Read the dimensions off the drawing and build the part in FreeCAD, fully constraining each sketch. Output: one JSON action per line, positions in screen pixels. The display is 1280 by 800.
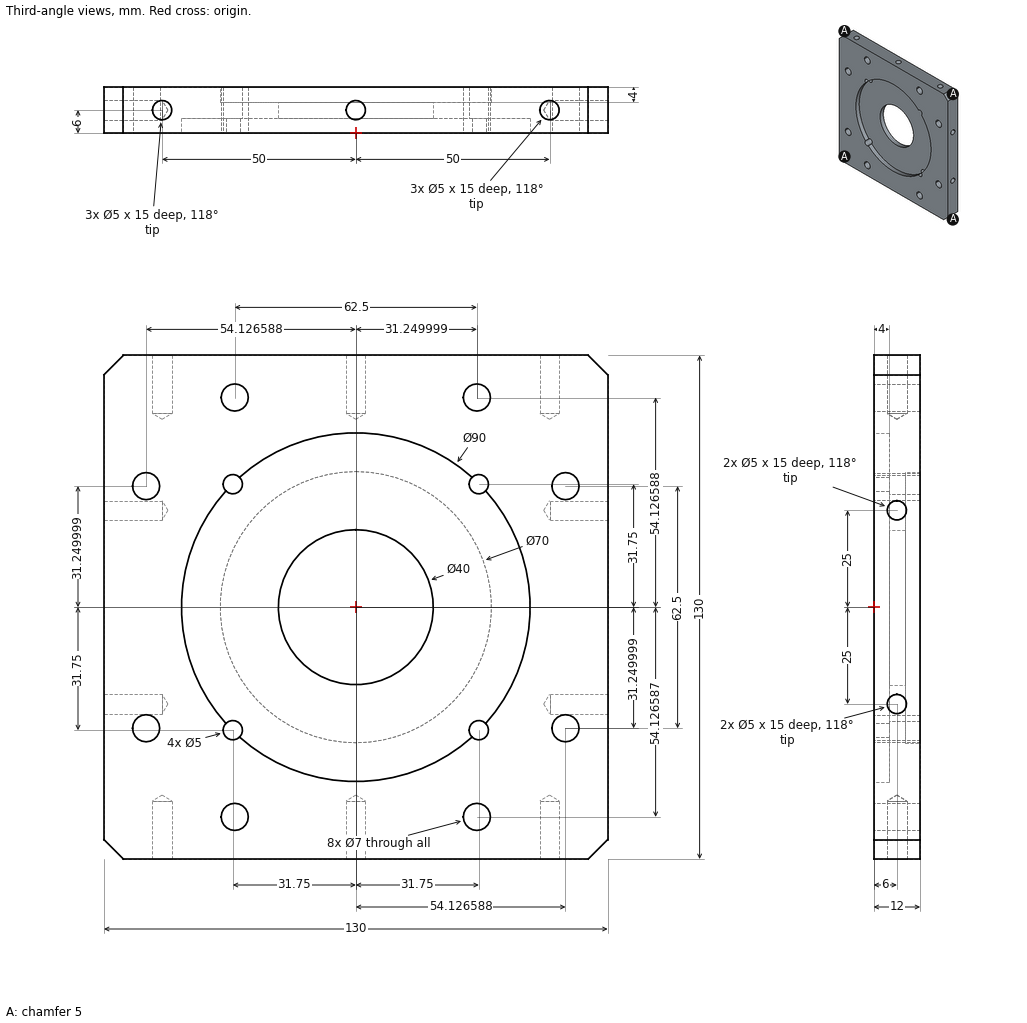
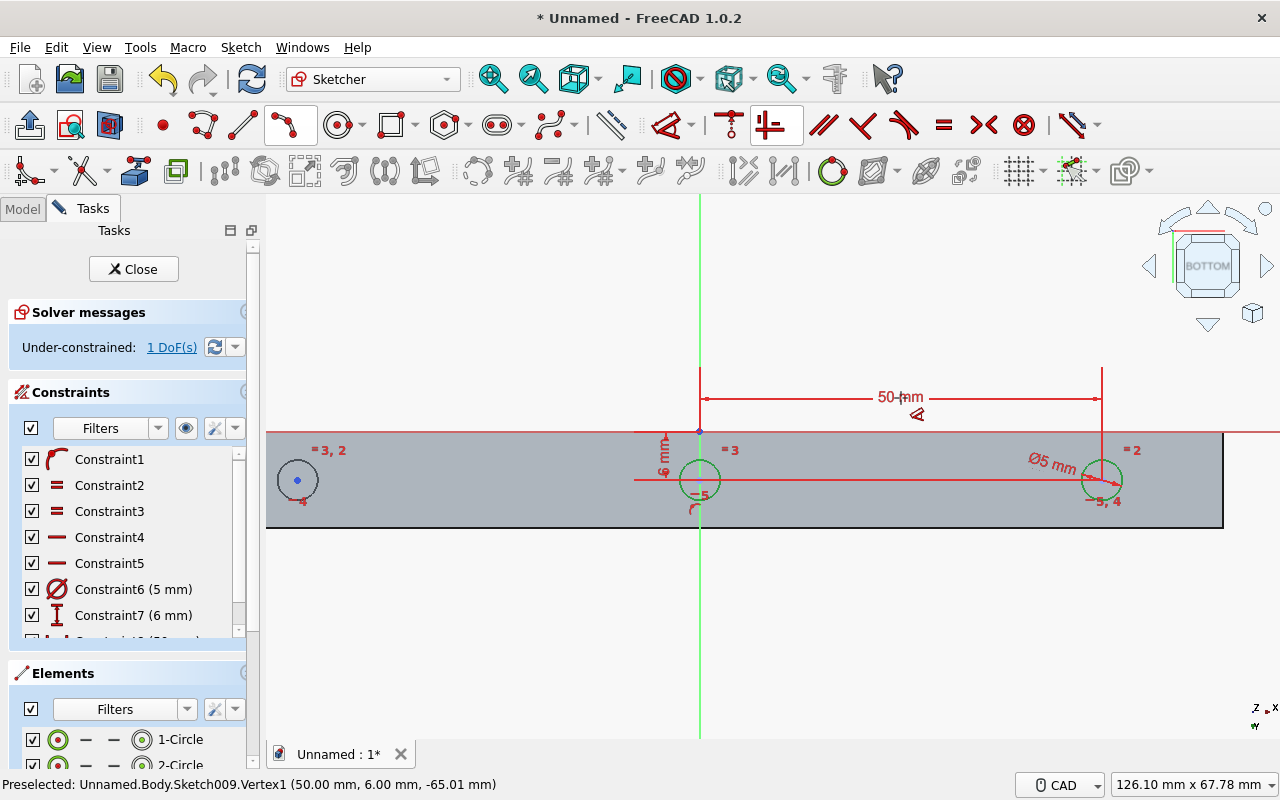
{"action": "left_click", "coordinate": [298, 480]}
{"action": "left_click", "coordinate": [499, 398]}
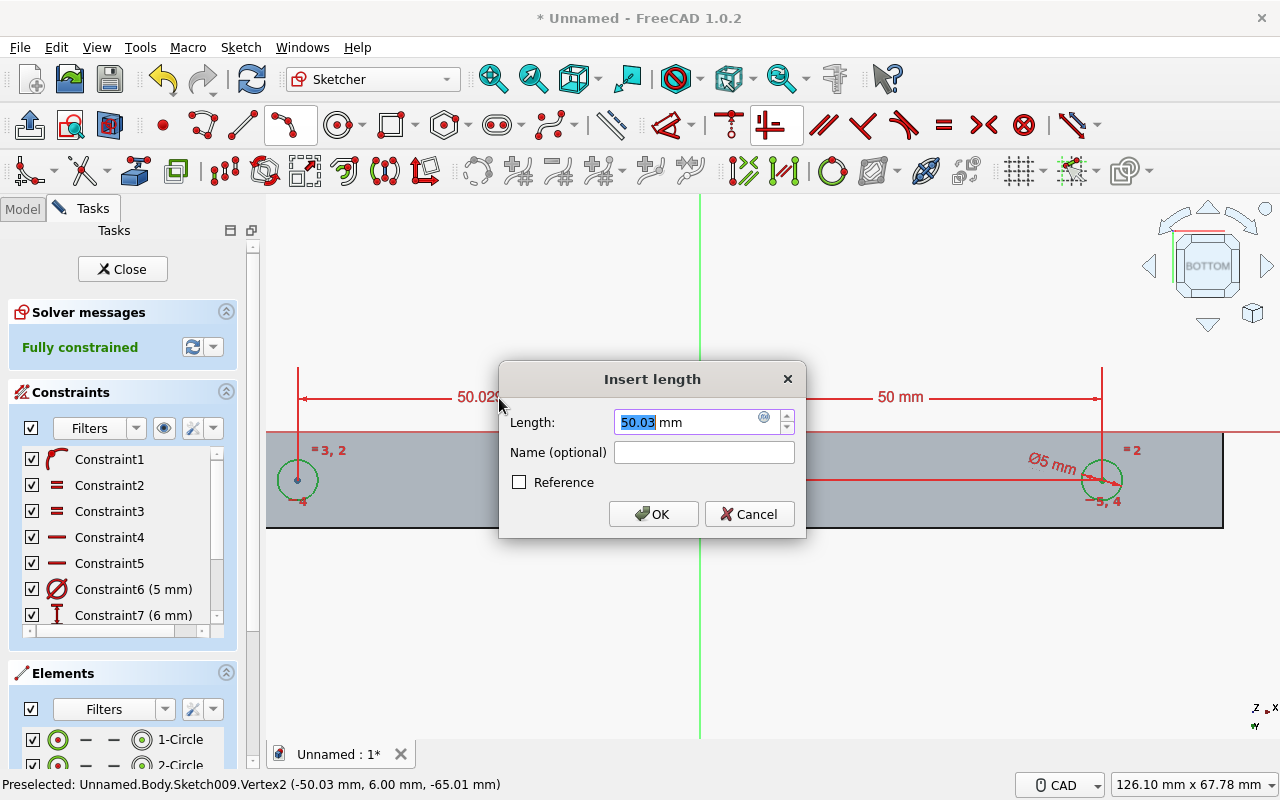
{"action": "type", "text": "50"}
{"action": "key", "text": "Return"}
{"action": "key", "text": "Escape"}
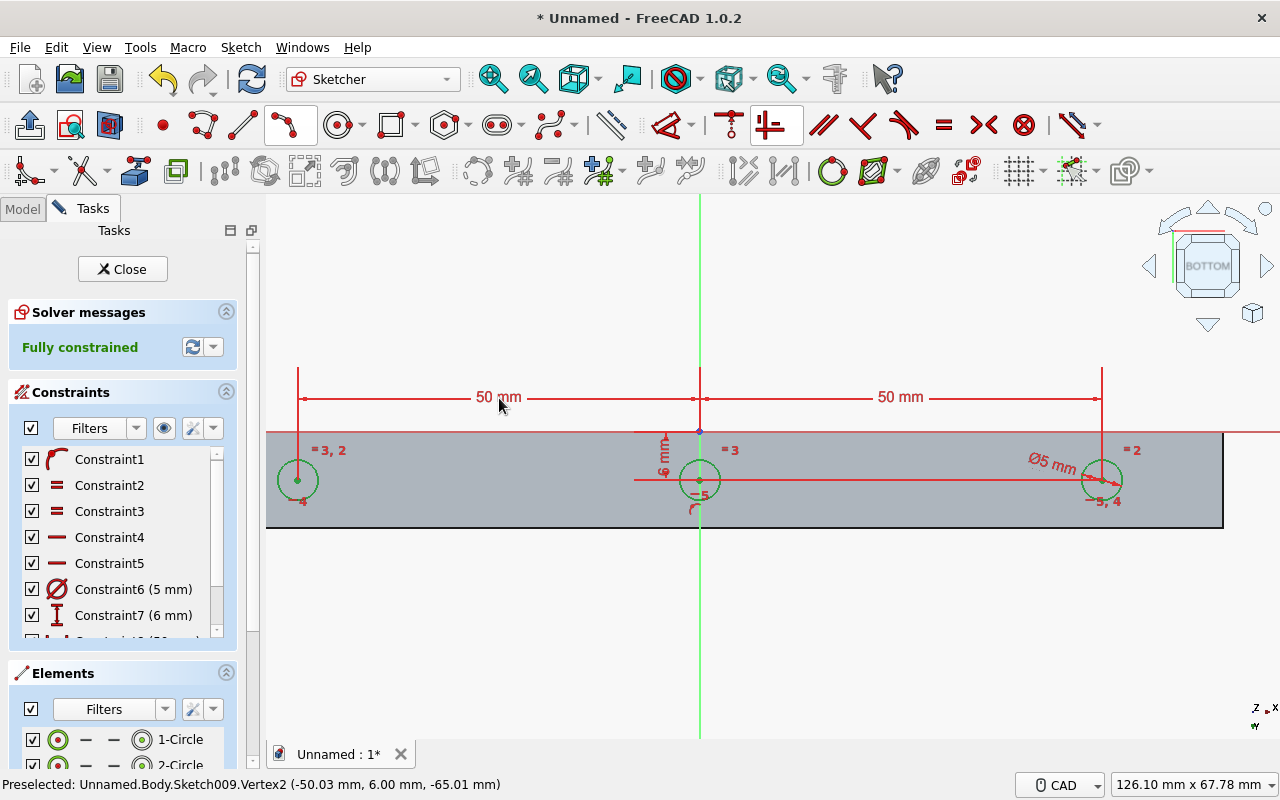
{"action": "left_click", "coordinate": [123, 269]}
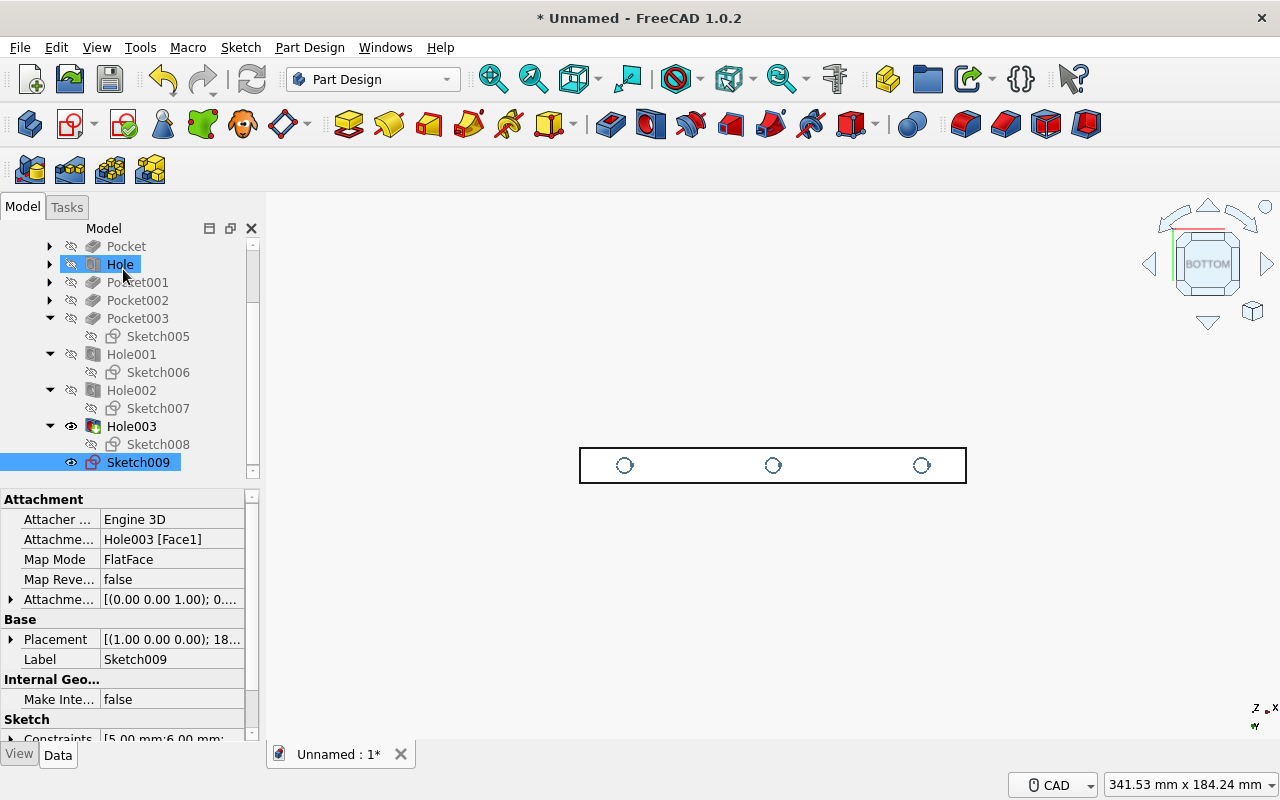
{"action": "left_click", "coordinate": [652, 124]}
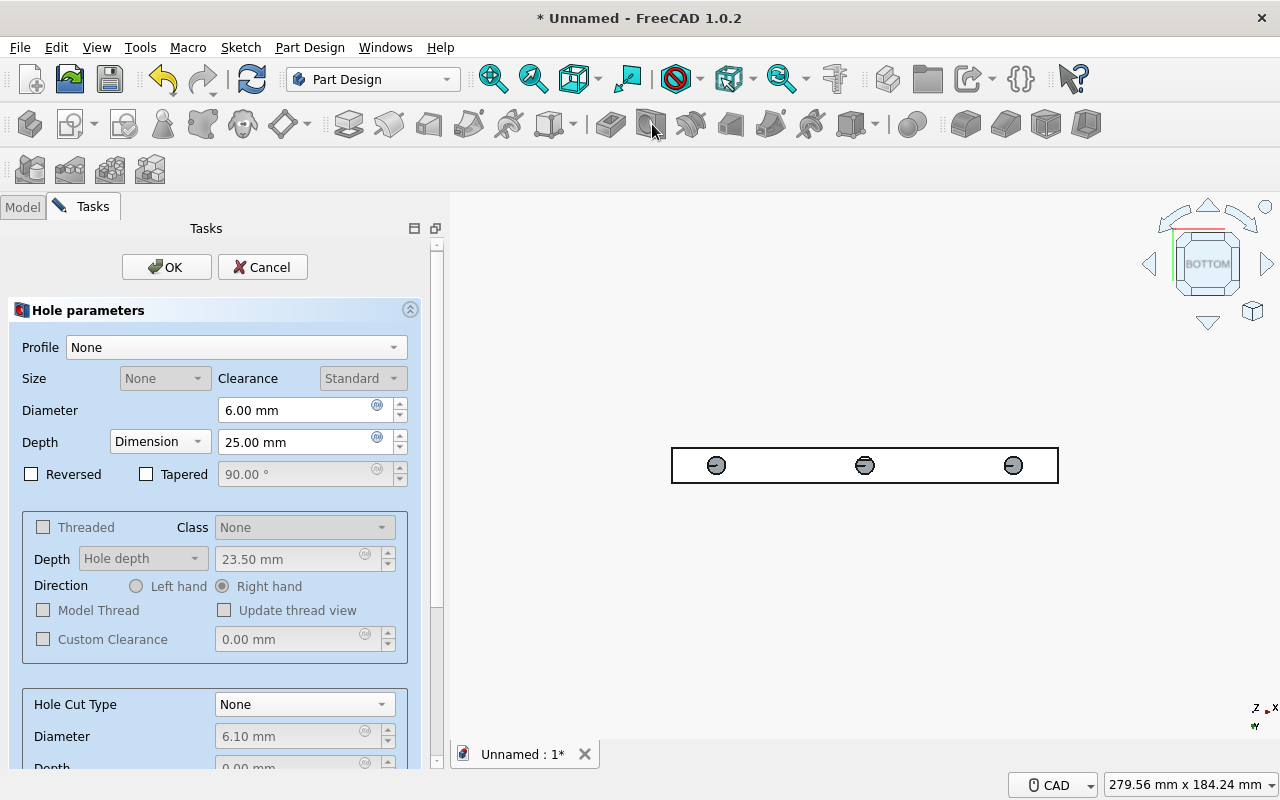
{"action": "triple_click", "coordinate": [305, 410]}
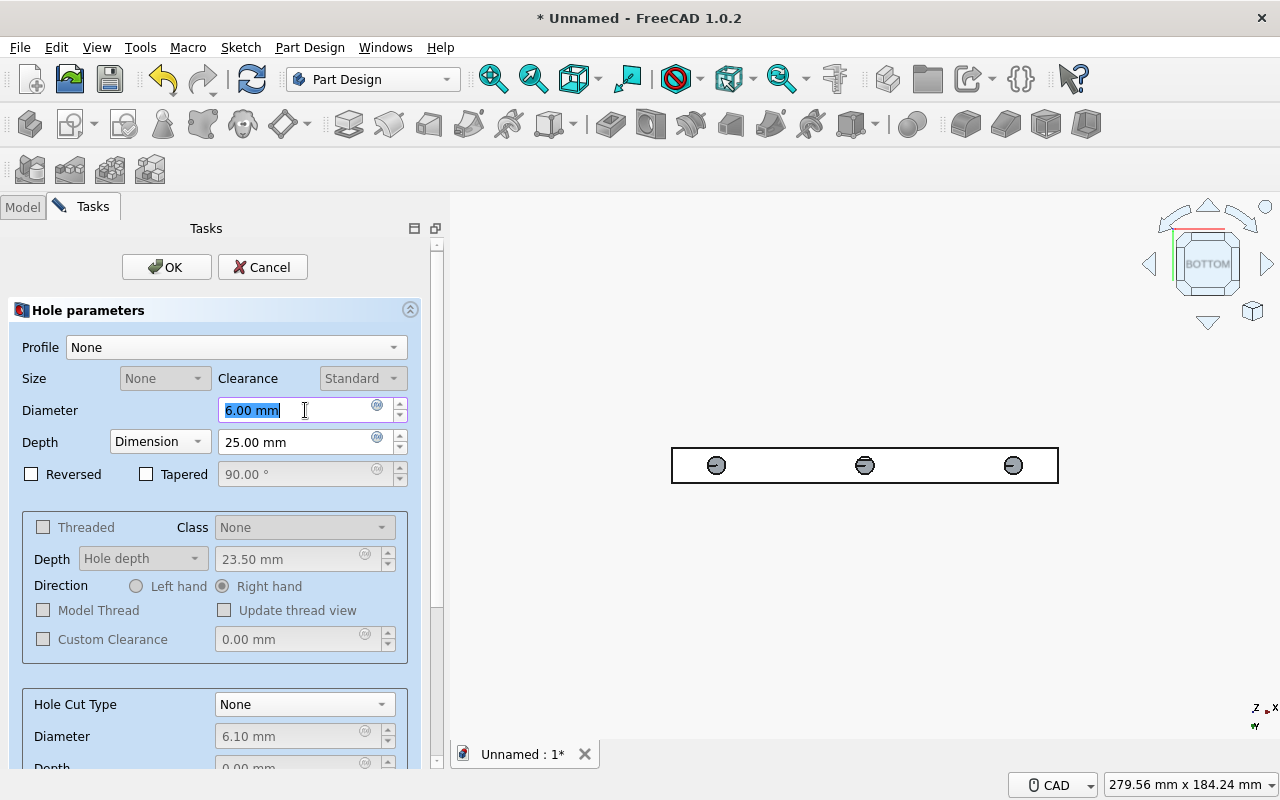
{"action": "type", "text": "5"}
{"action": "key", "text": "Tab"}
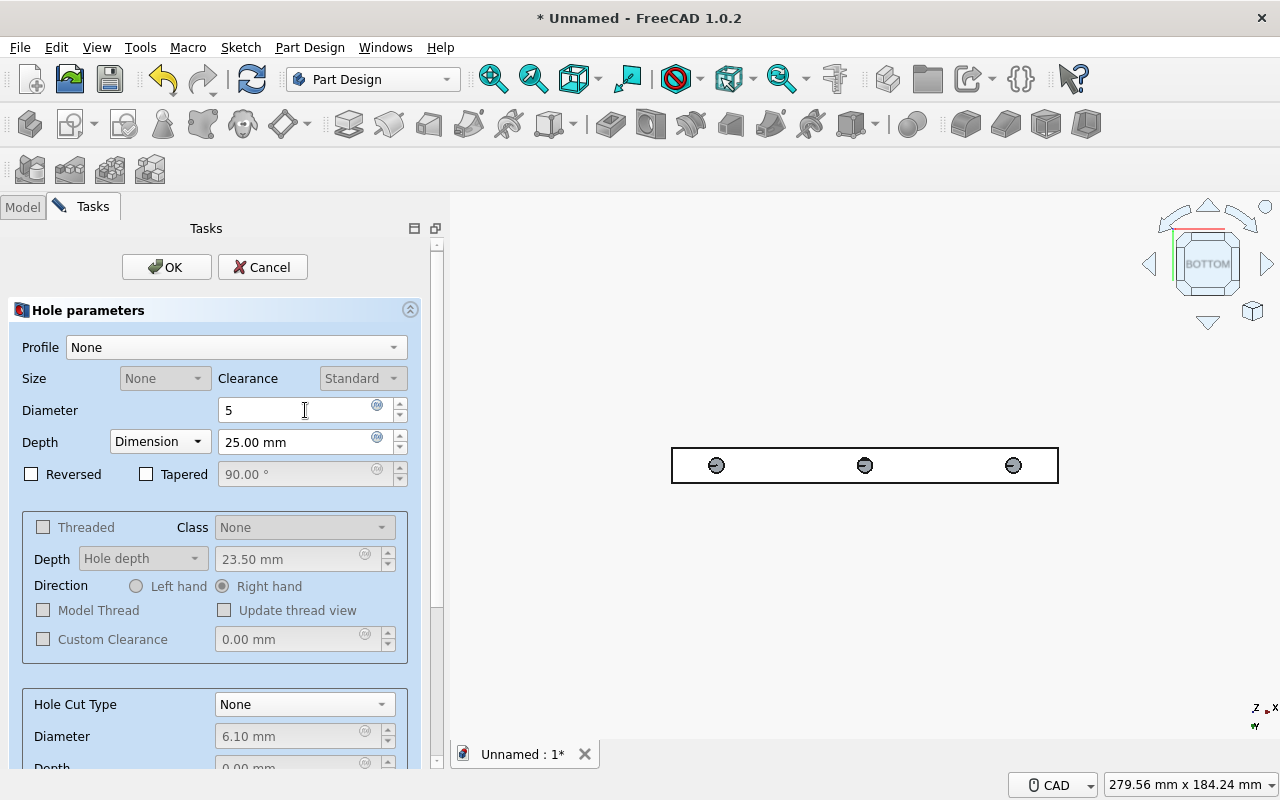
{"action": "triple_click", "coordinate": [305, 442]}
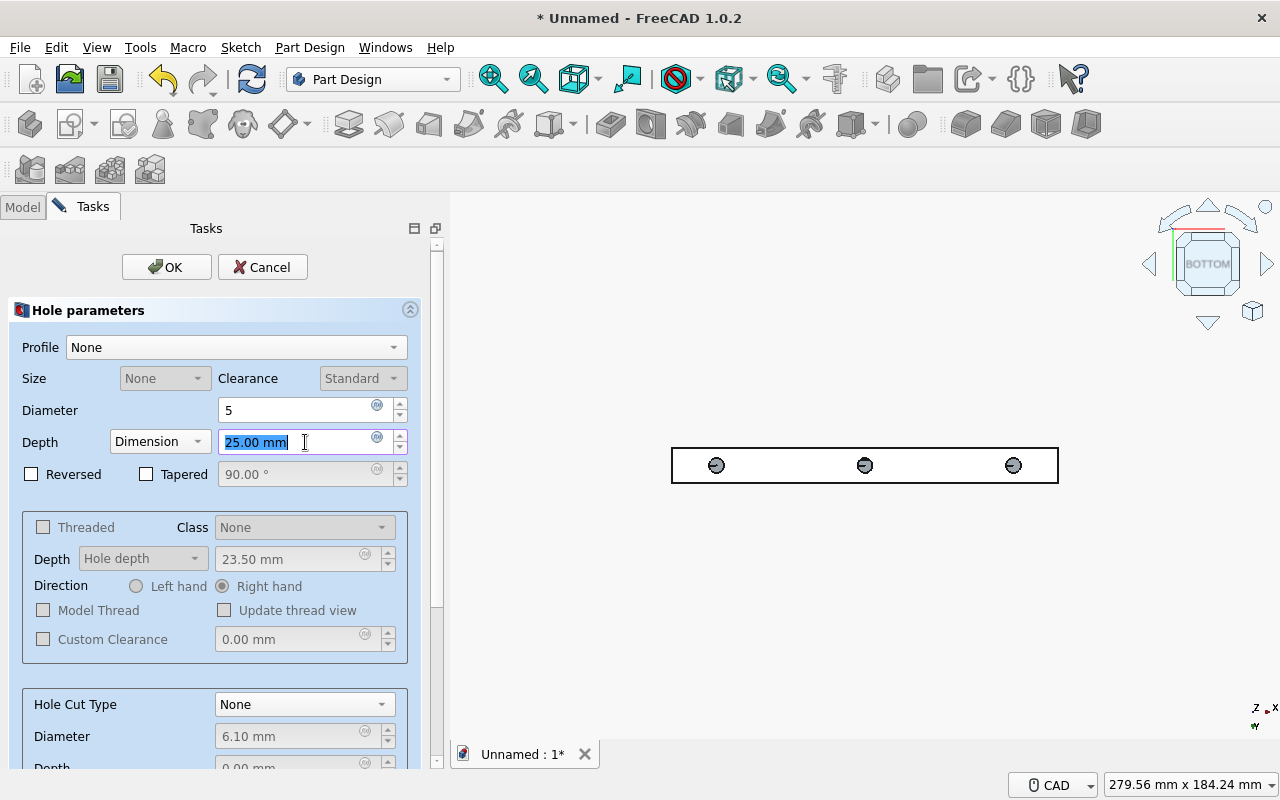
{"action": "type", "text": "15"}
{"action": "key", "text": "Tab"}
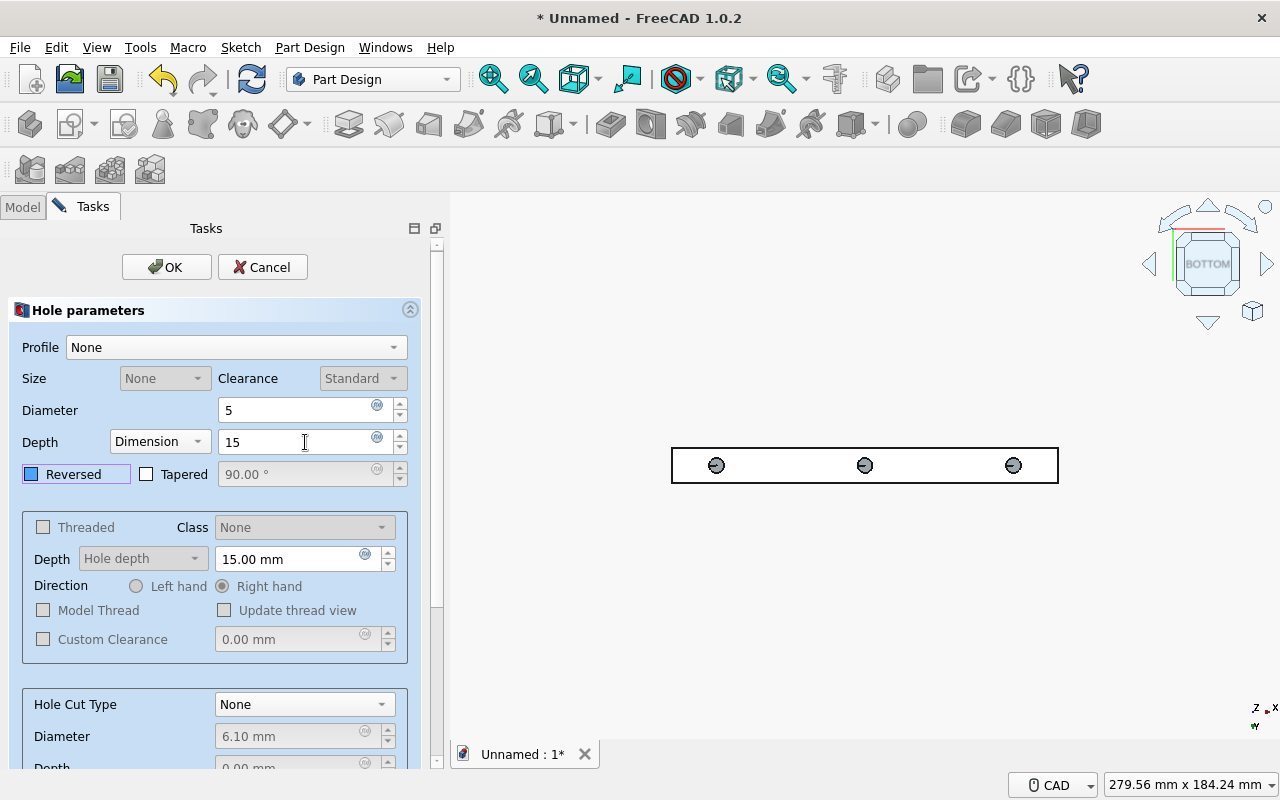
{"action": "left_click", "coordinate": [167, 267]}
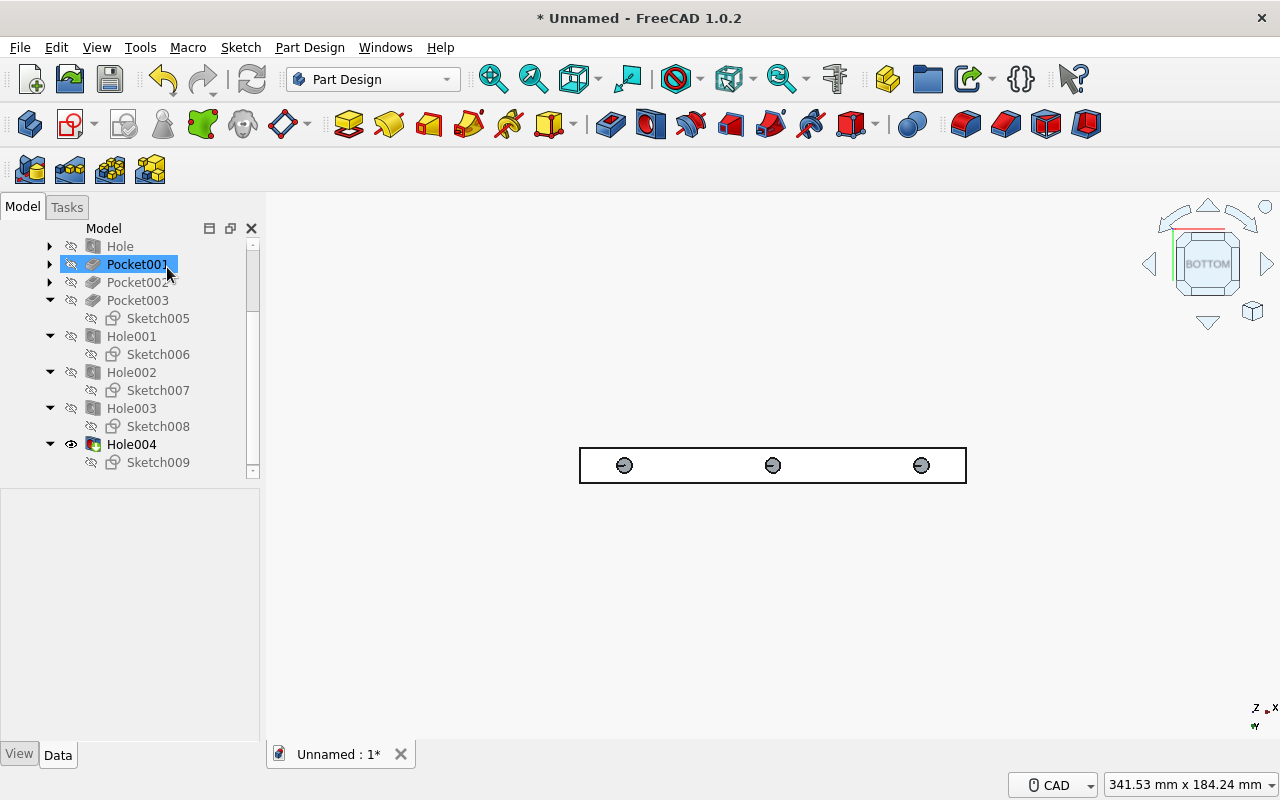
{"action": "key", "text": "v f"}